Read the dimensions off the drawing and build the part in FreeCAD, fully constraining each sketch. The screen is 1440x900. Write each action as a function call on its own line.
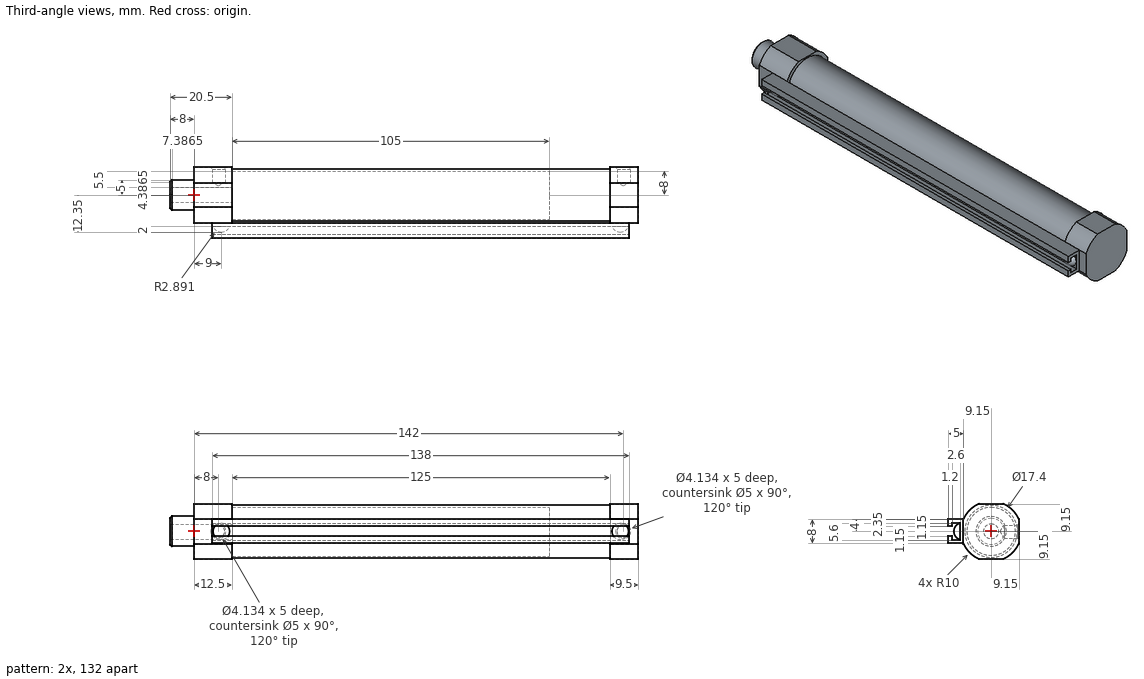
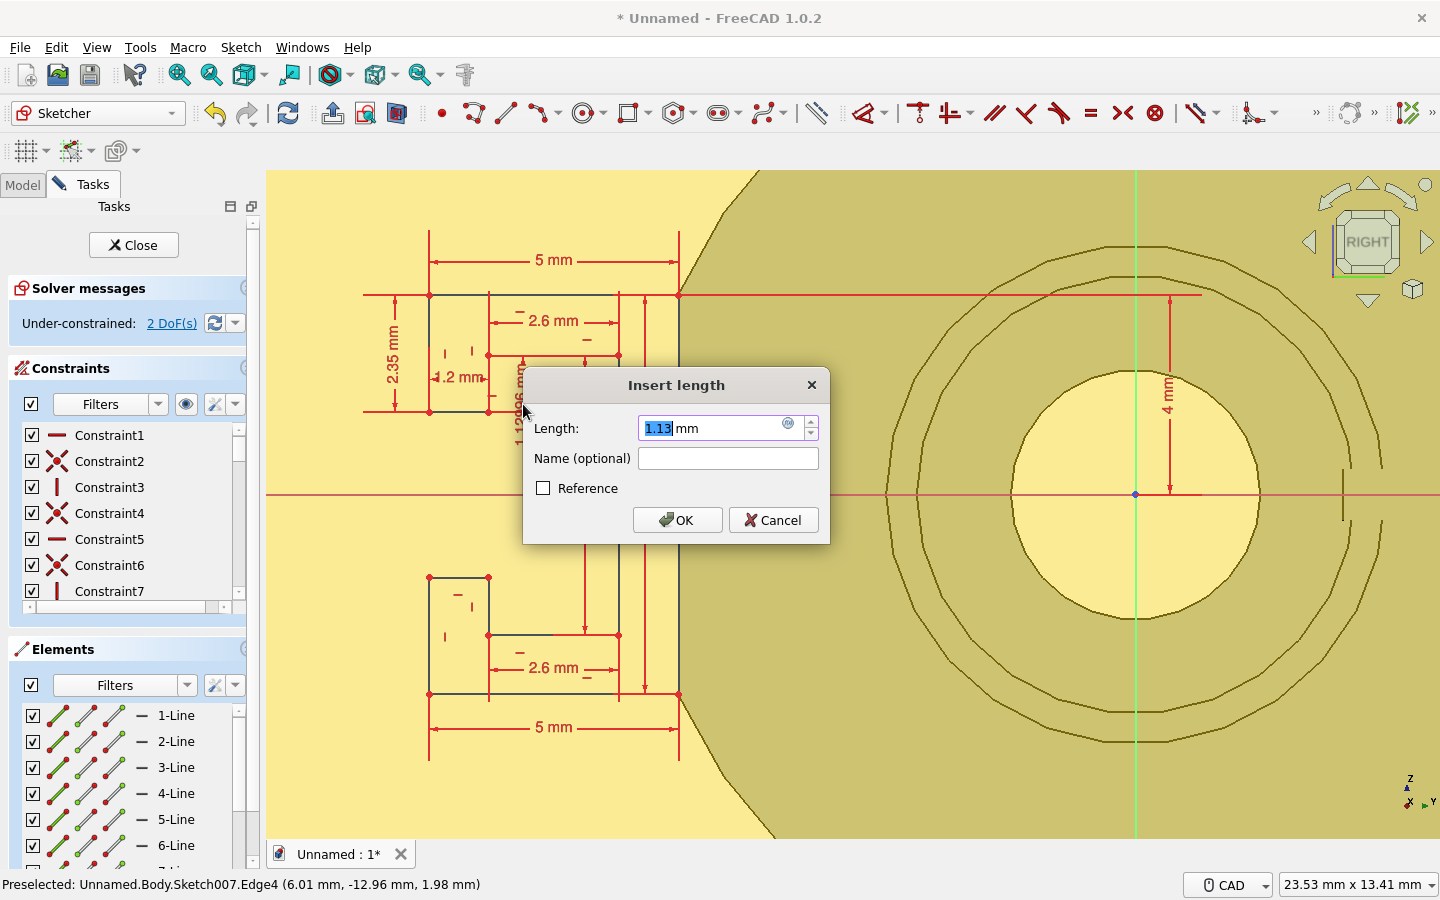
text(1.15)
key(Return)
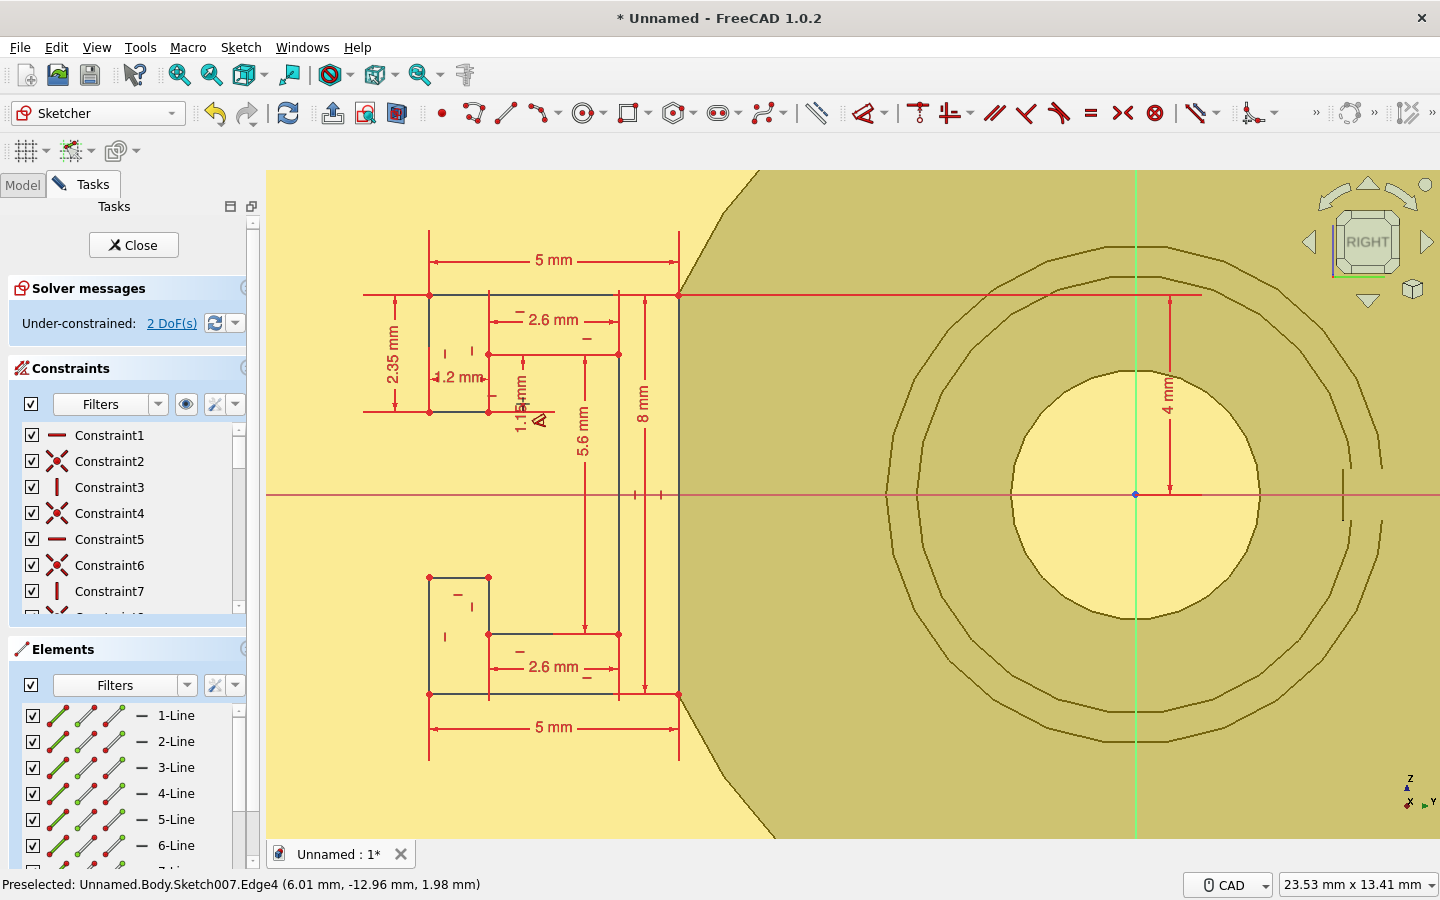
click(489, 618)
click(455, 606)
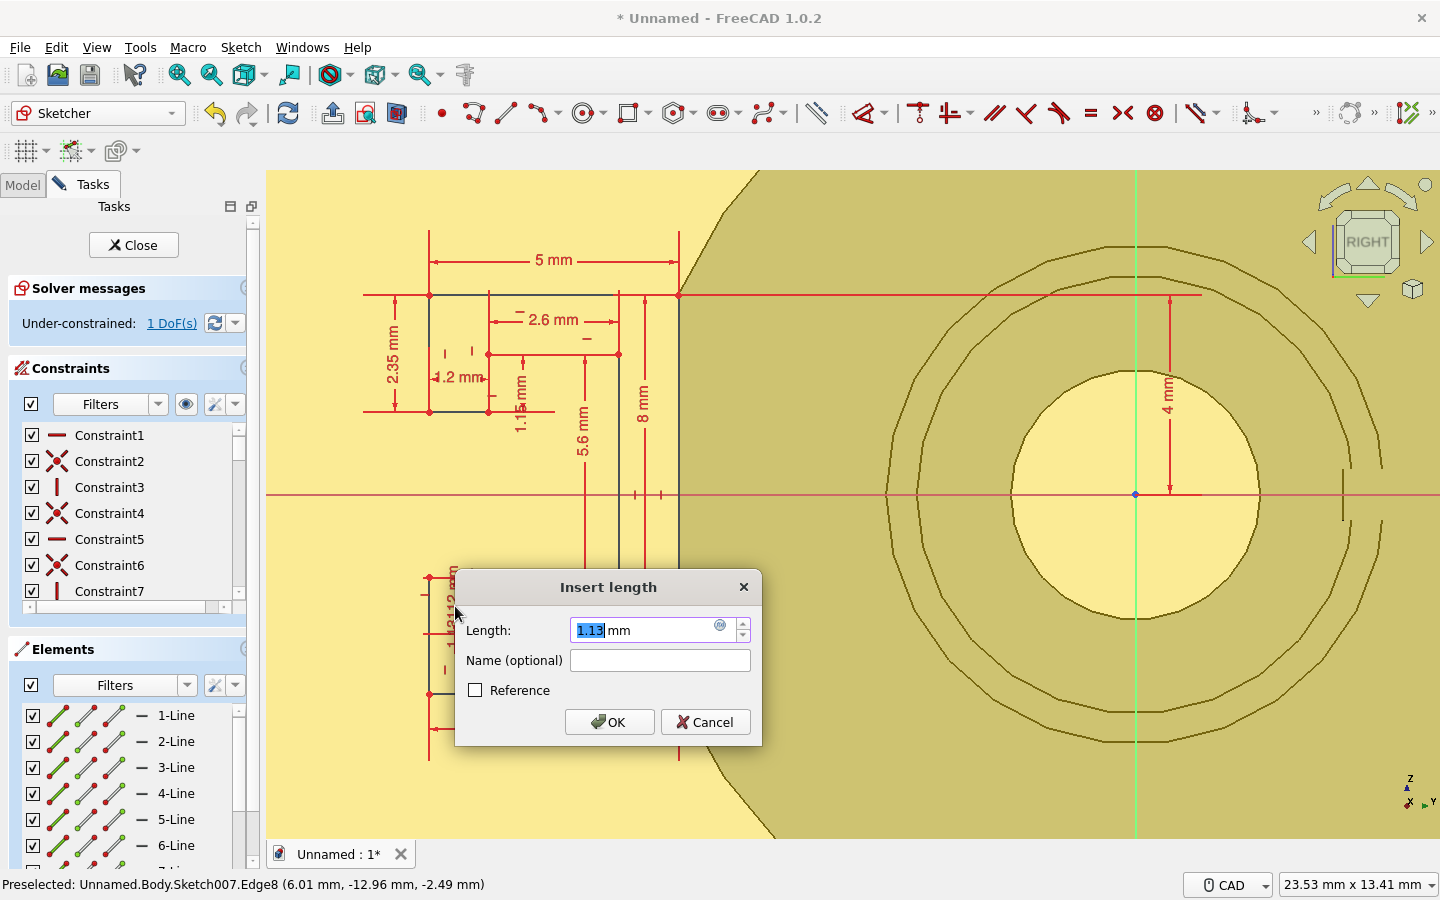
text(1.15)
key(Return)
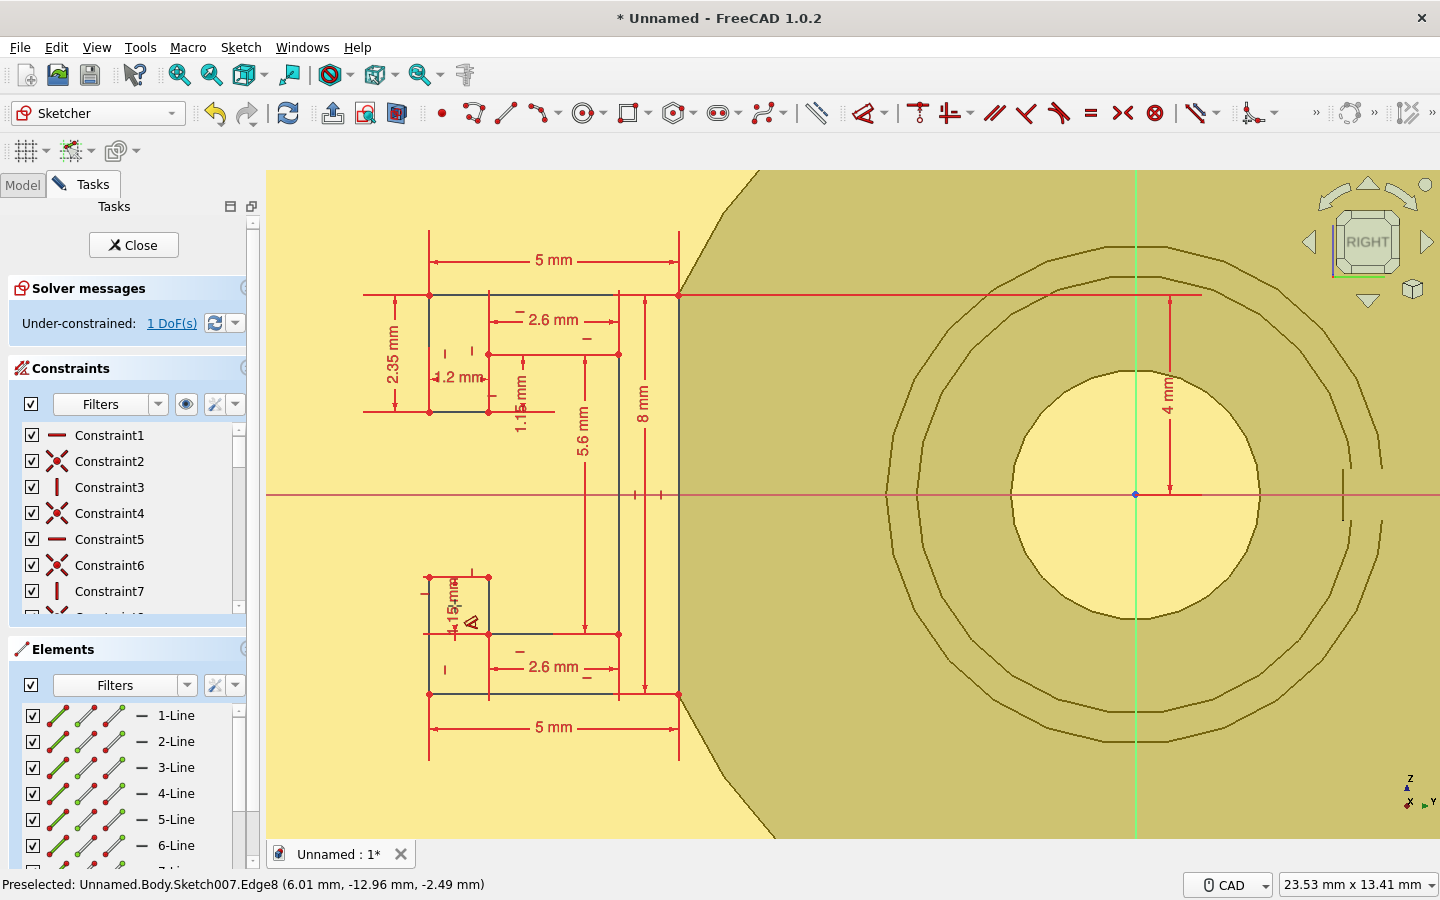
click(679, 295)
click(907, 261)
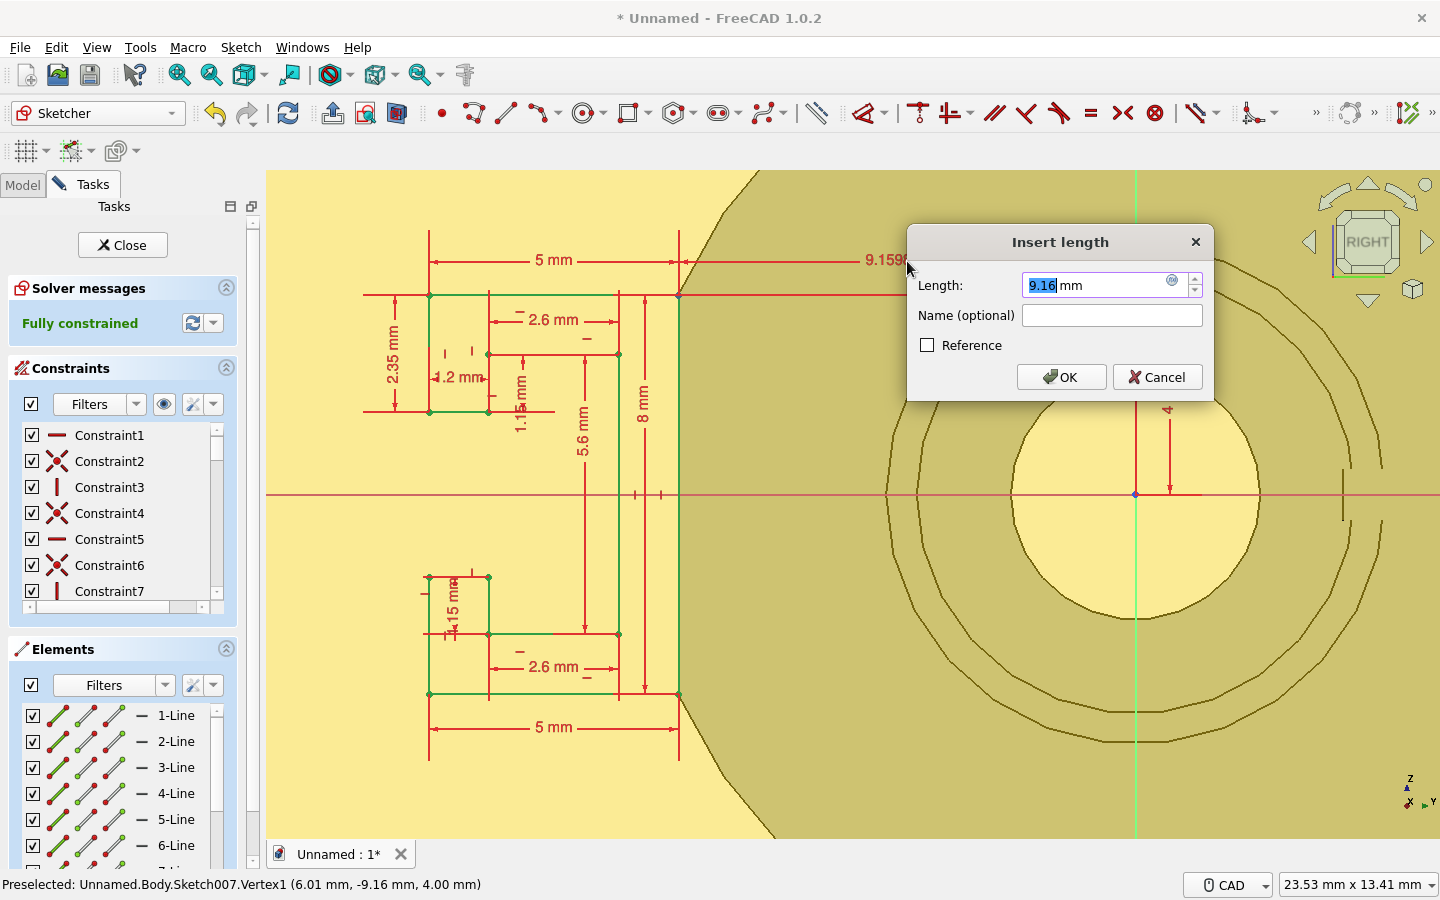
text(9.15)
key(Return)
key(Escape)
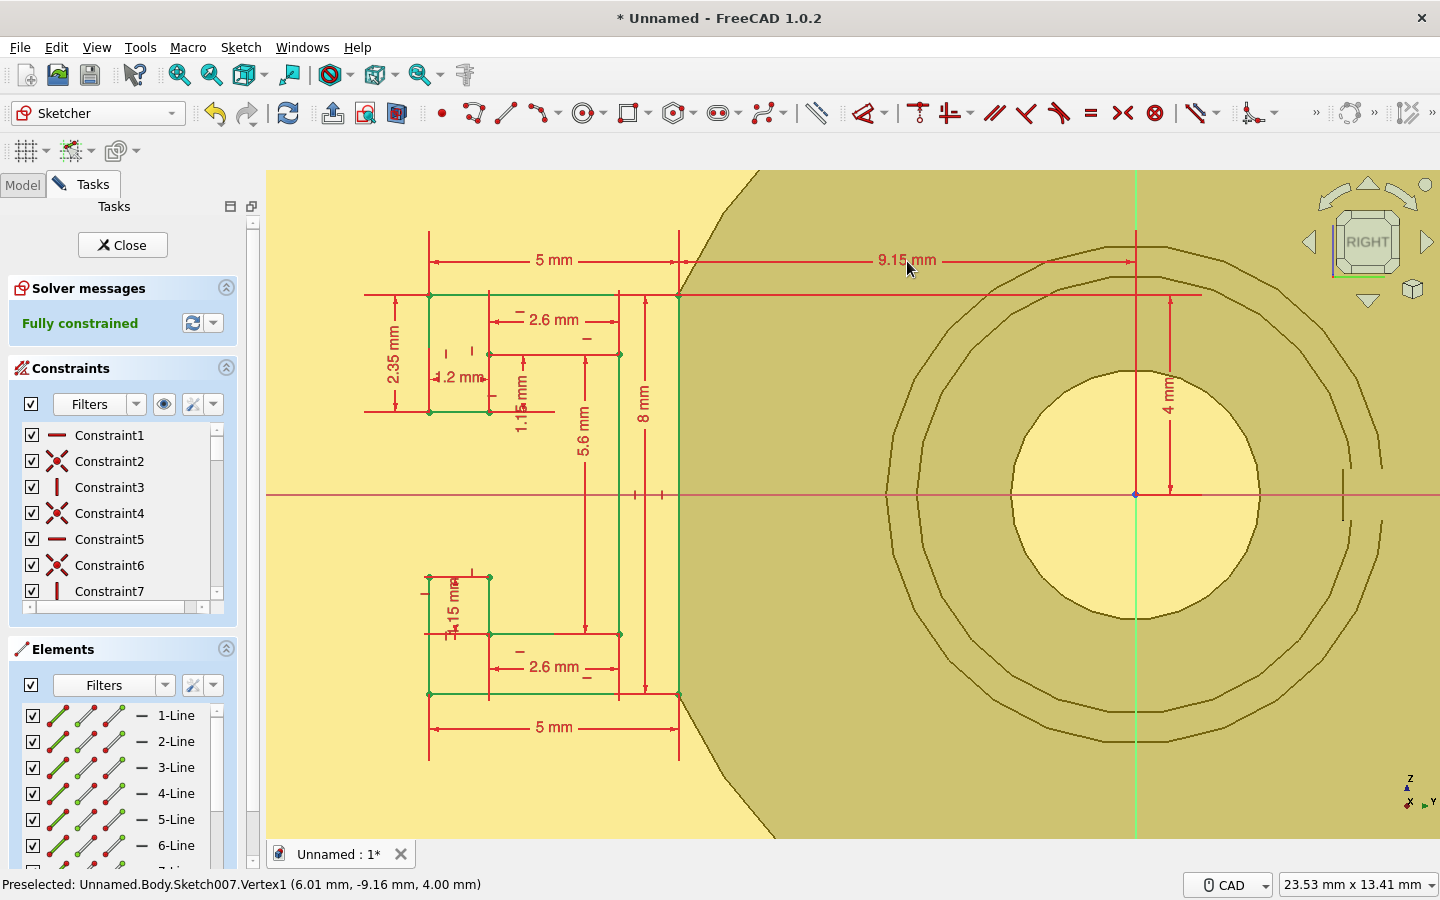
click(123, 245)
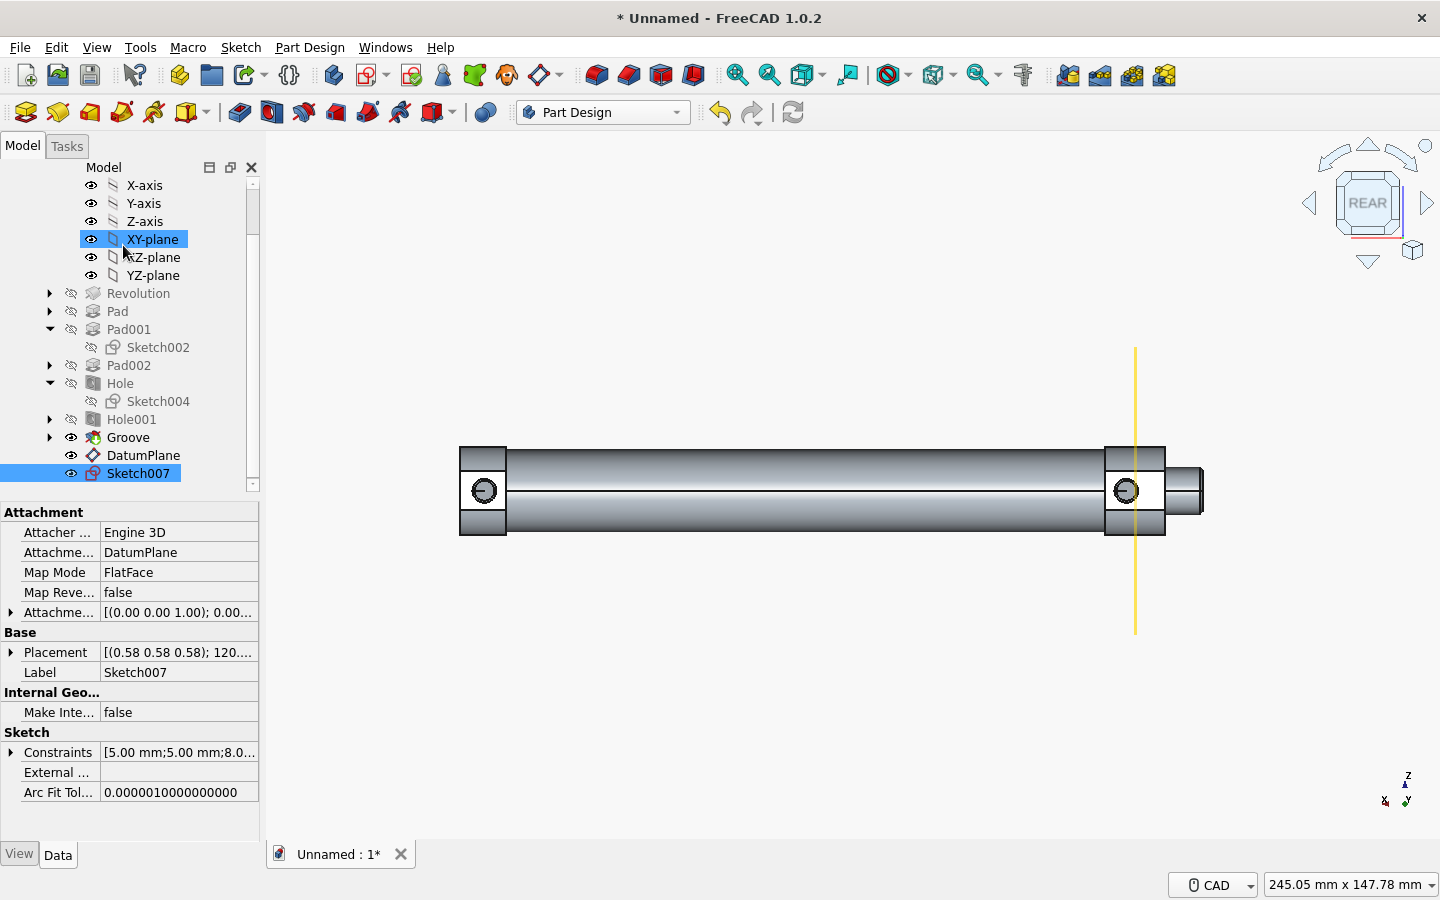
click(26, 112)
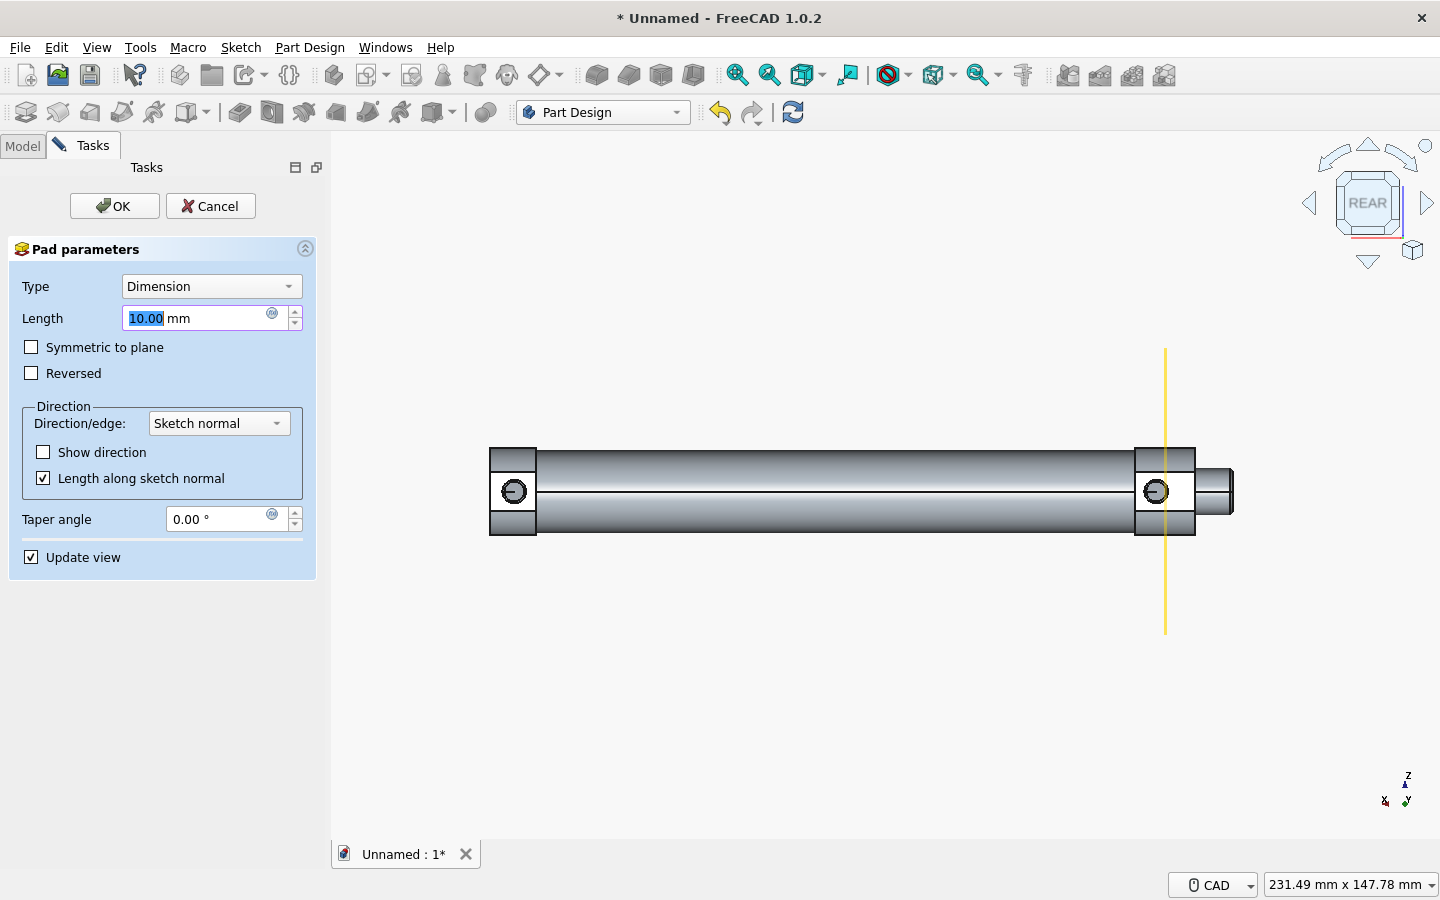
text(138)
key(Tab)